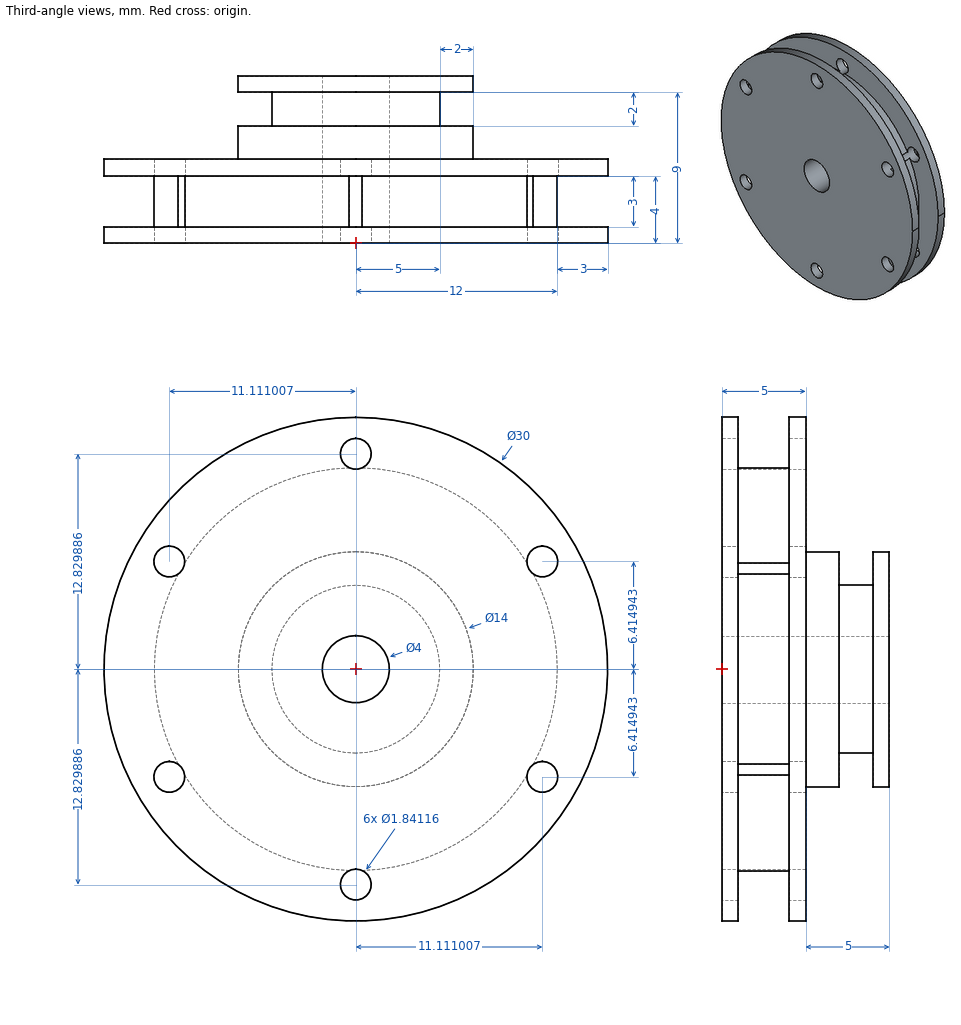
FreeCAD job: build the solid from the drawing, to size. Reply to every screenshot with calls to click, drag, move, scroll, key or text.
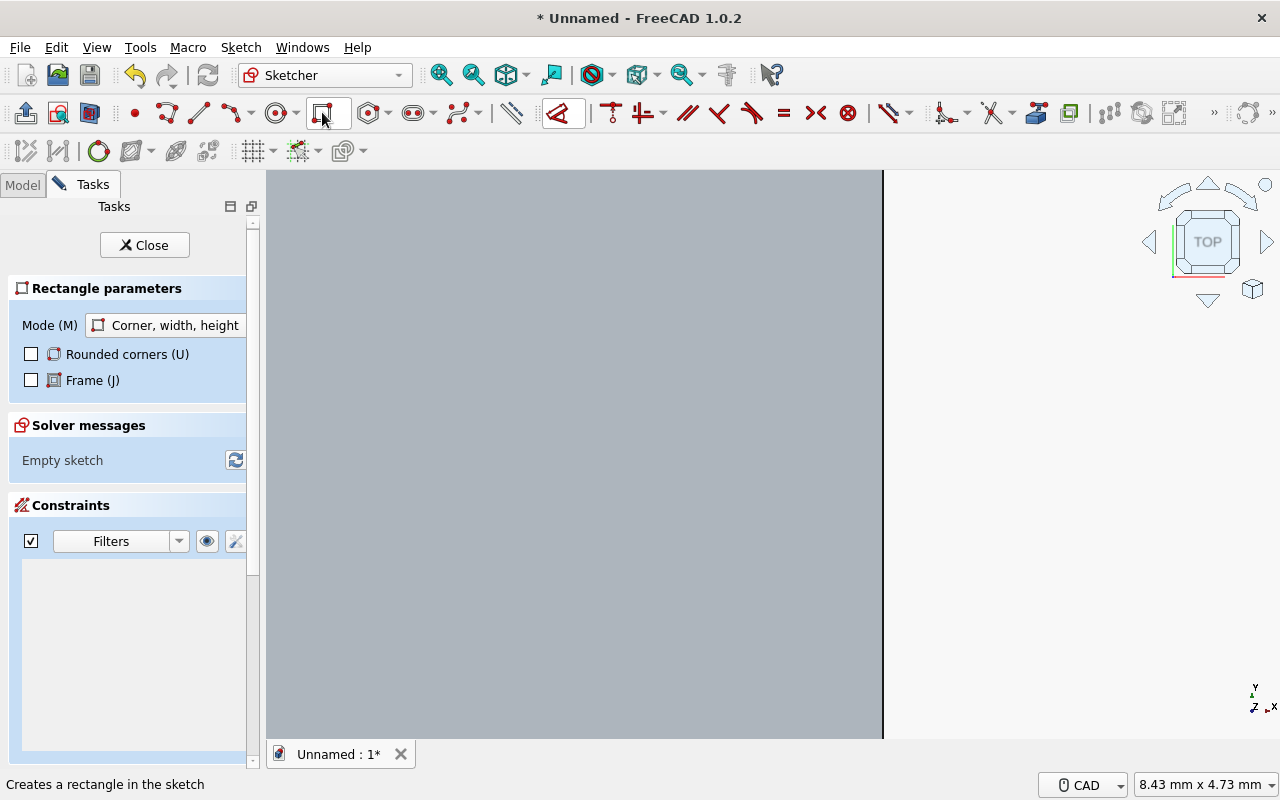
click(522, 266)
move(883, 627)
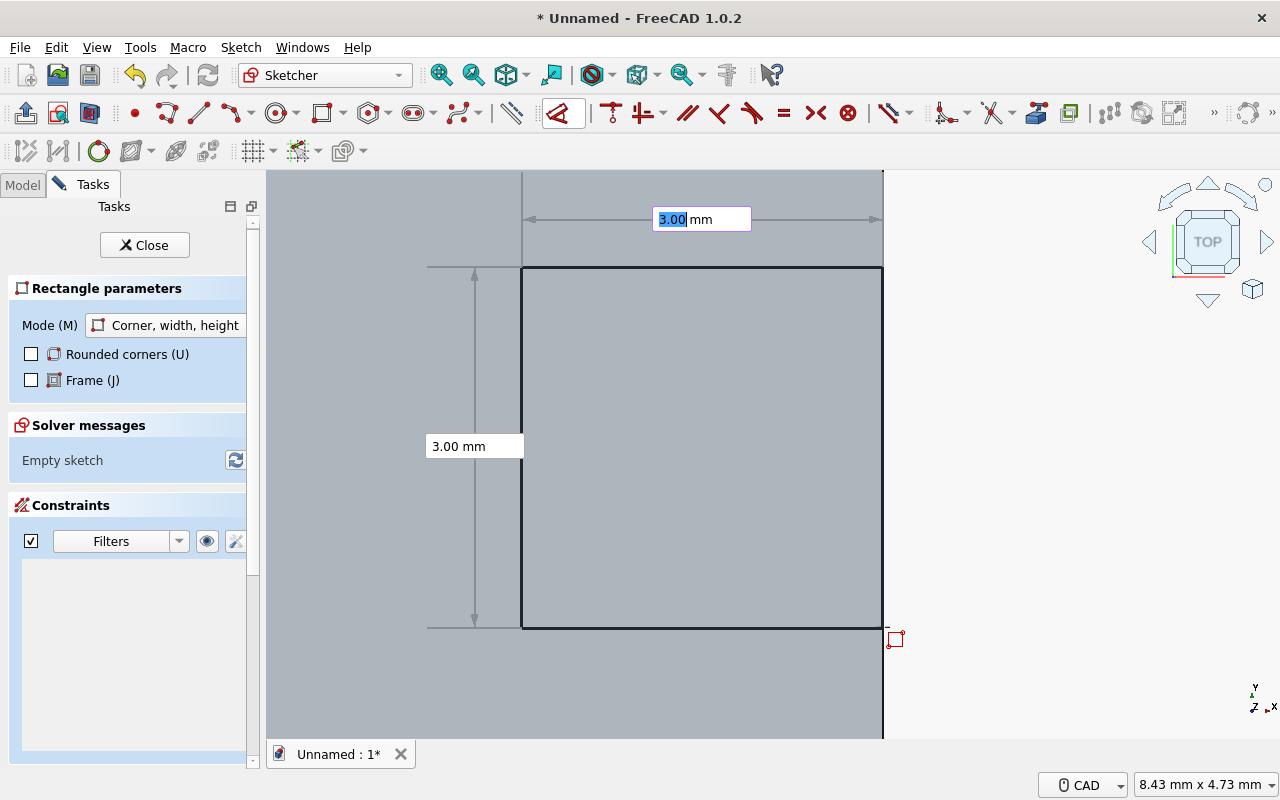
text(3)
key(Tab)
text(3)
key(Return)
key(Escape)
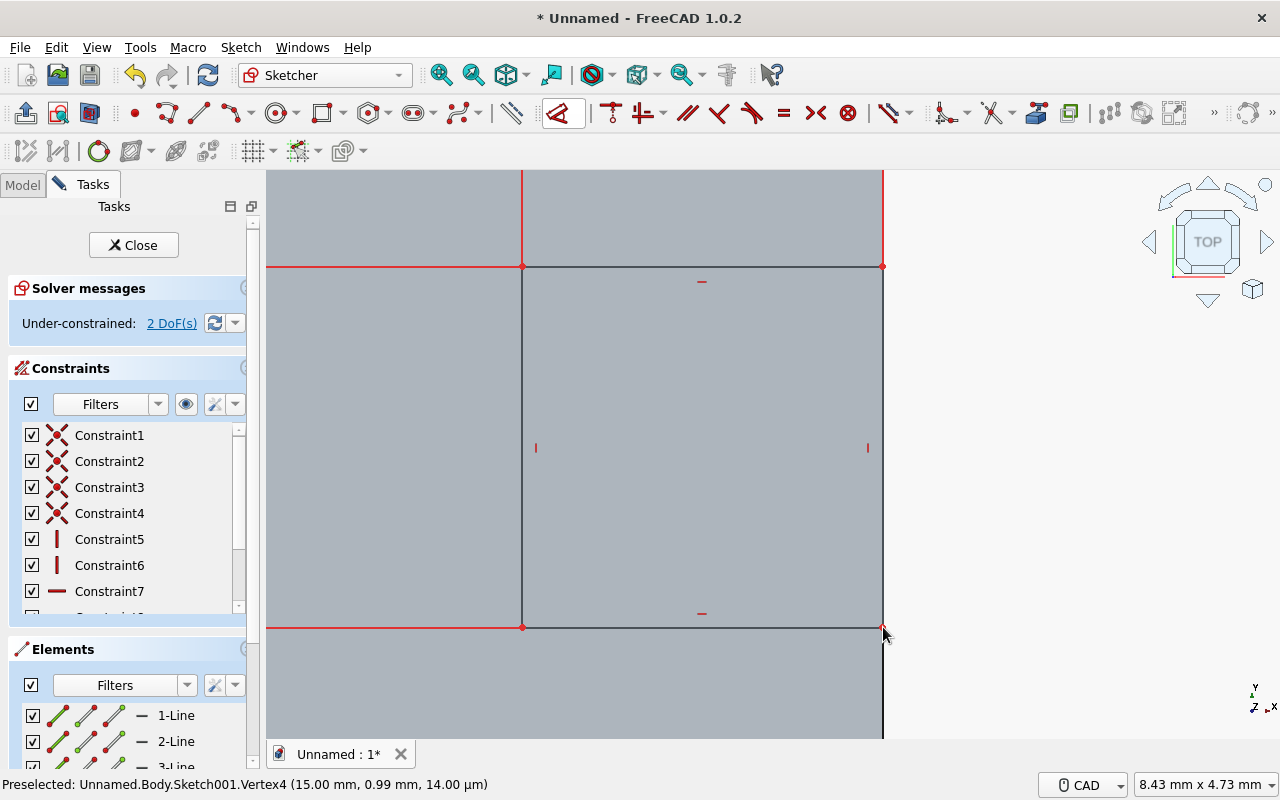
click(558, 114)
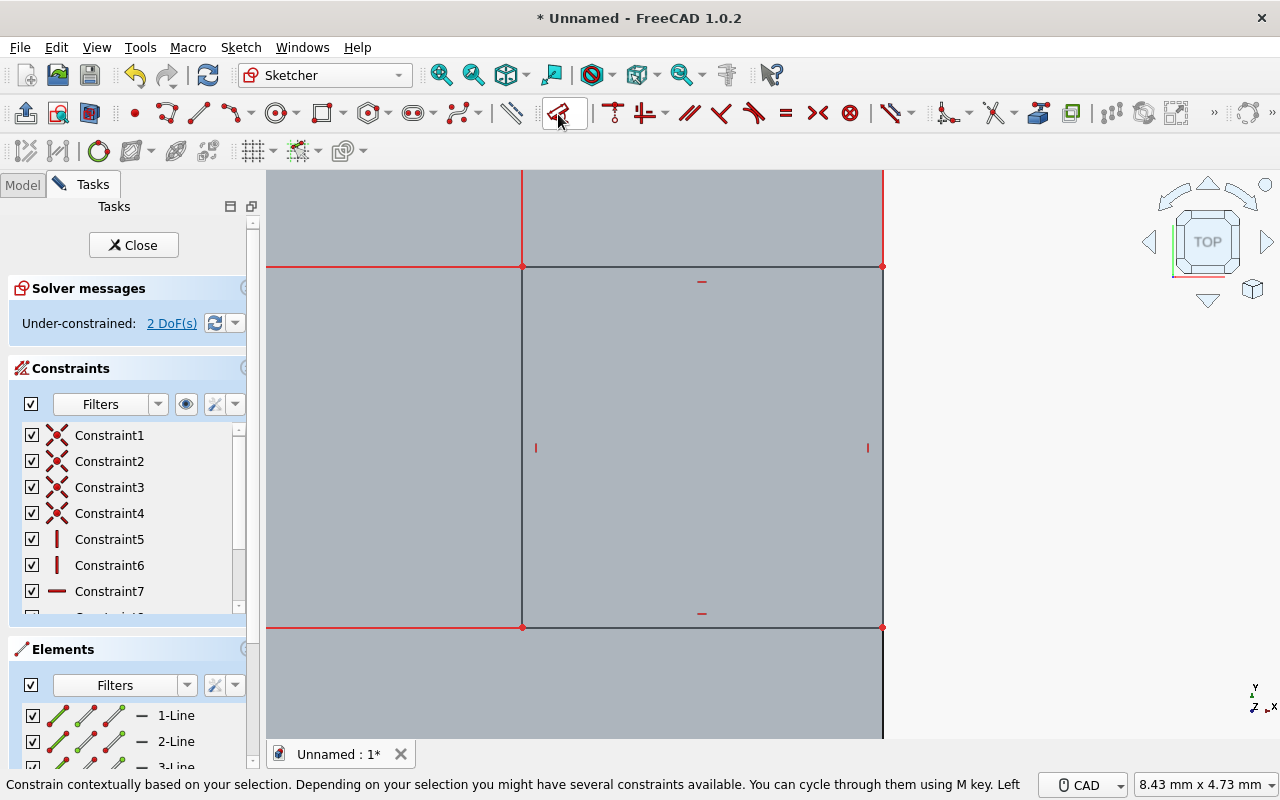
click(522, 267)
click(556, 489)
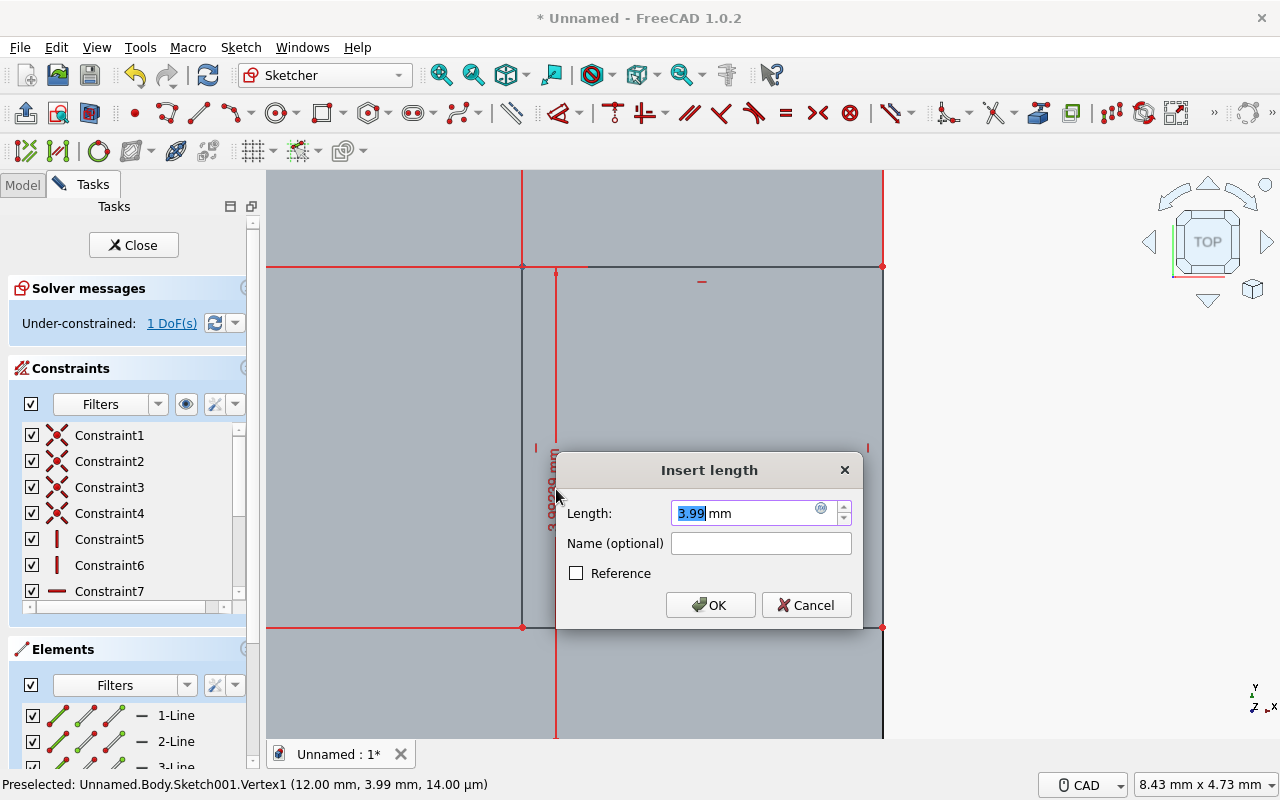
text(4)
key(Return)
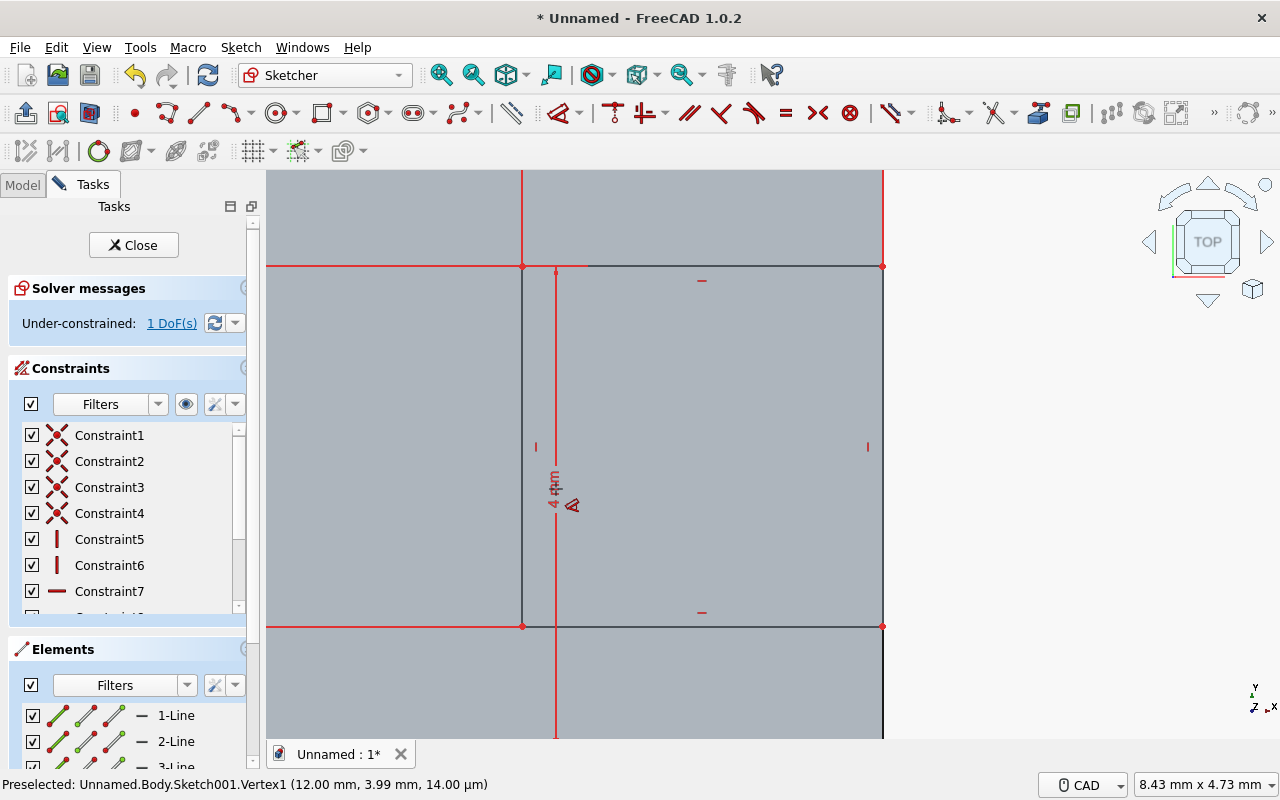
click(522, 266)
click(408, 232)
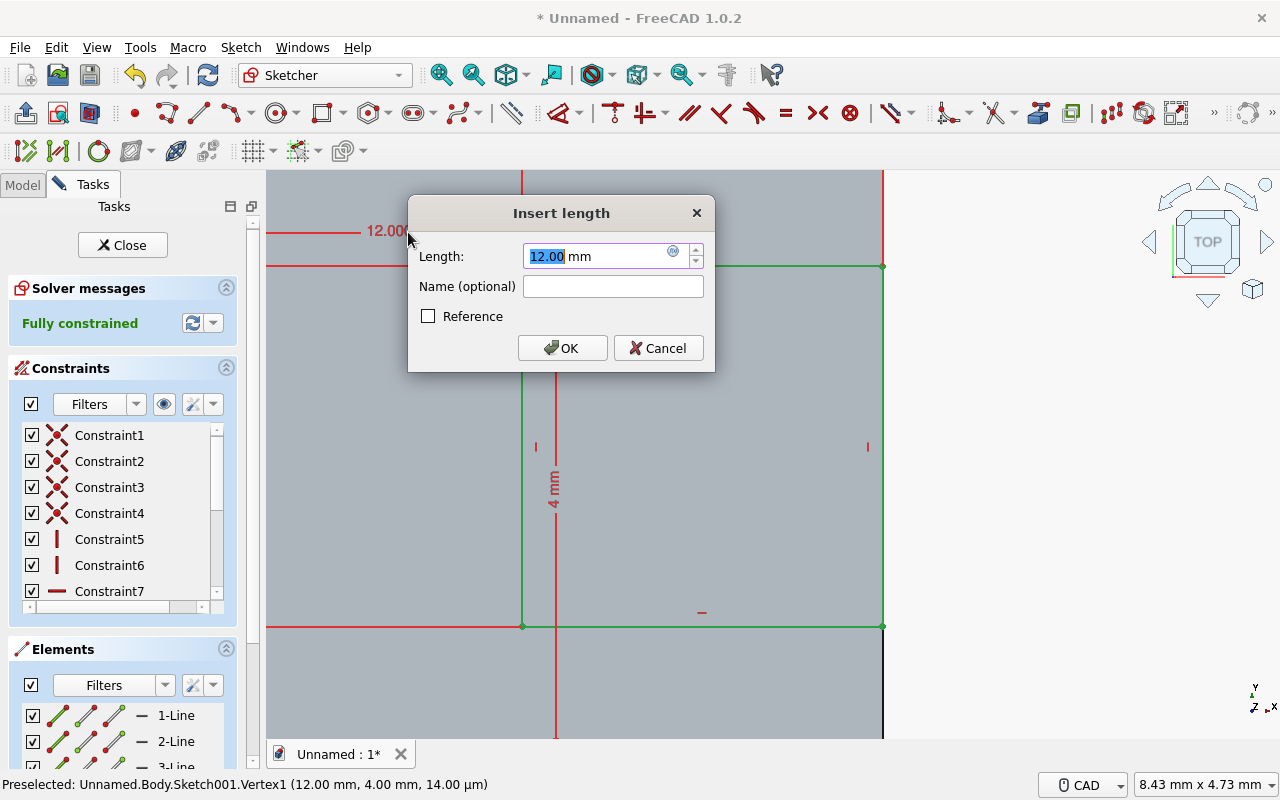
text(12)
key(Return)
key(Escape)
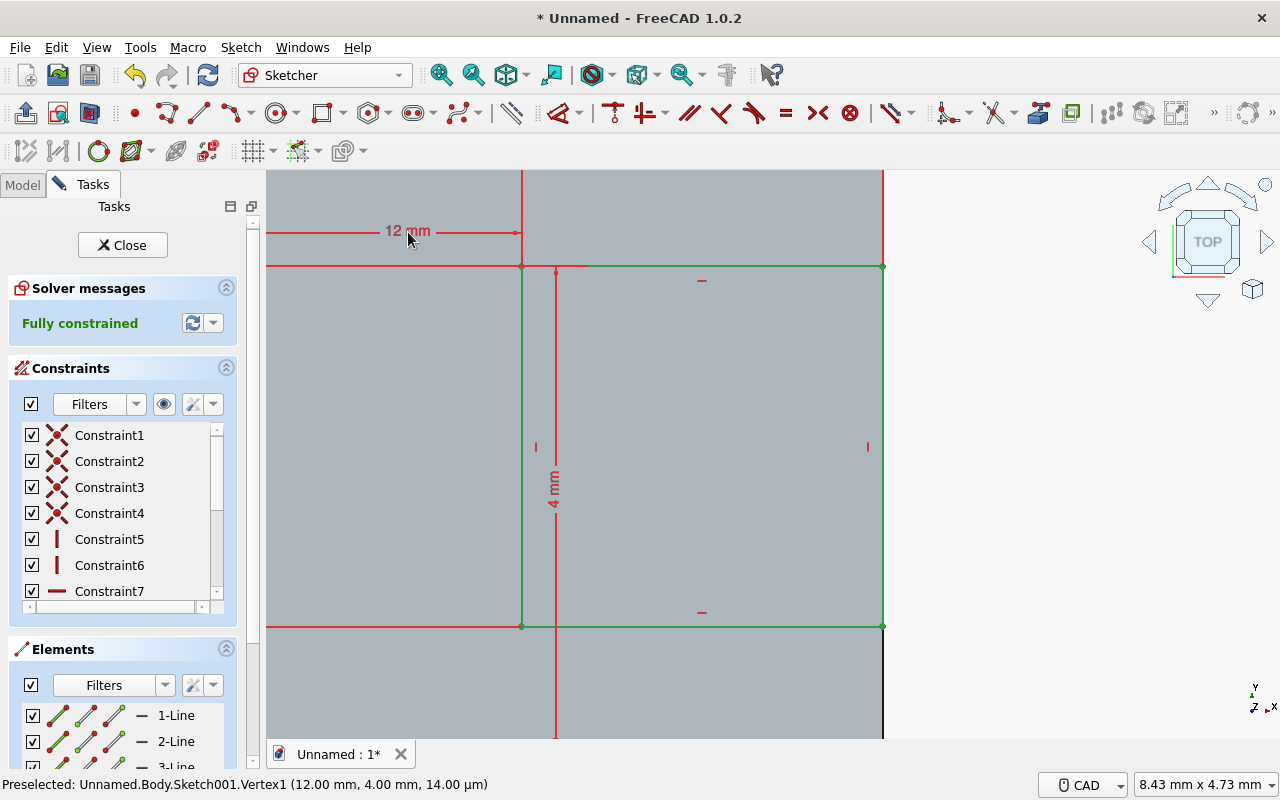
click(123, 245)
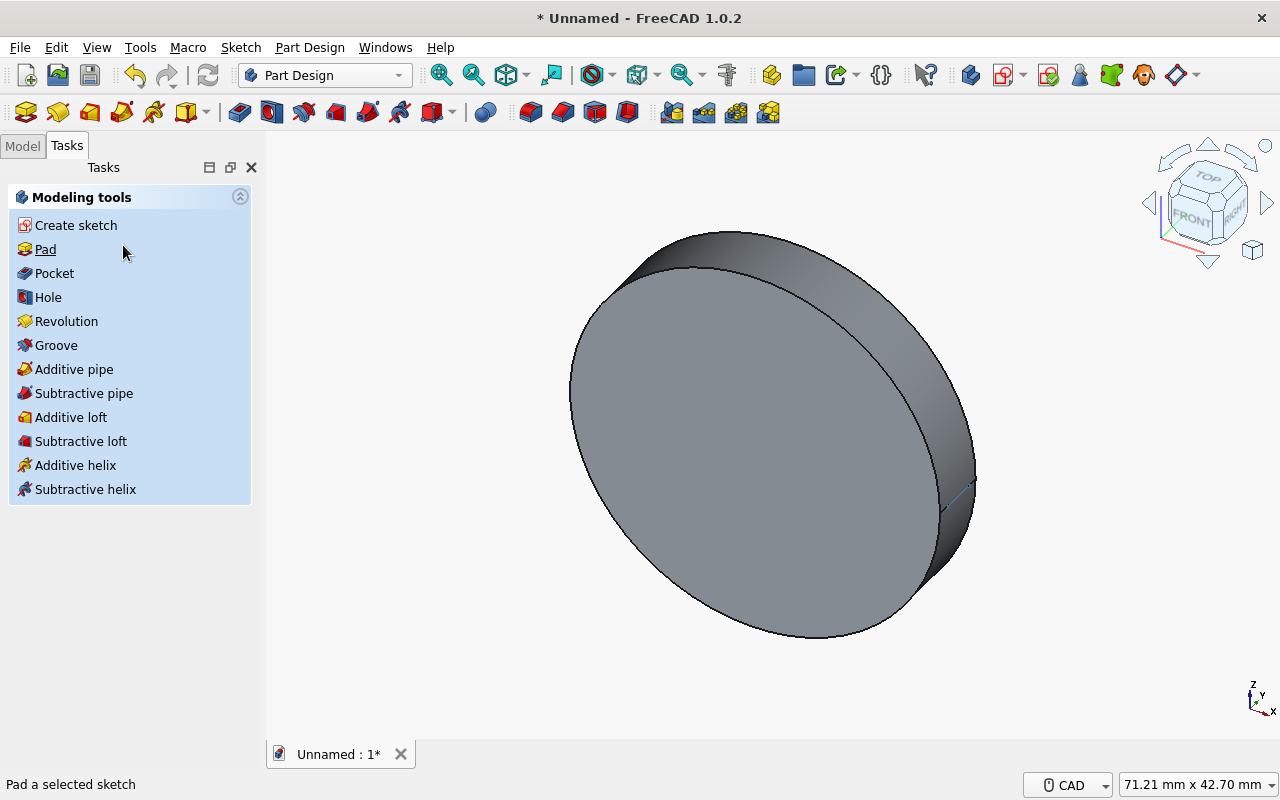
click(304, 112)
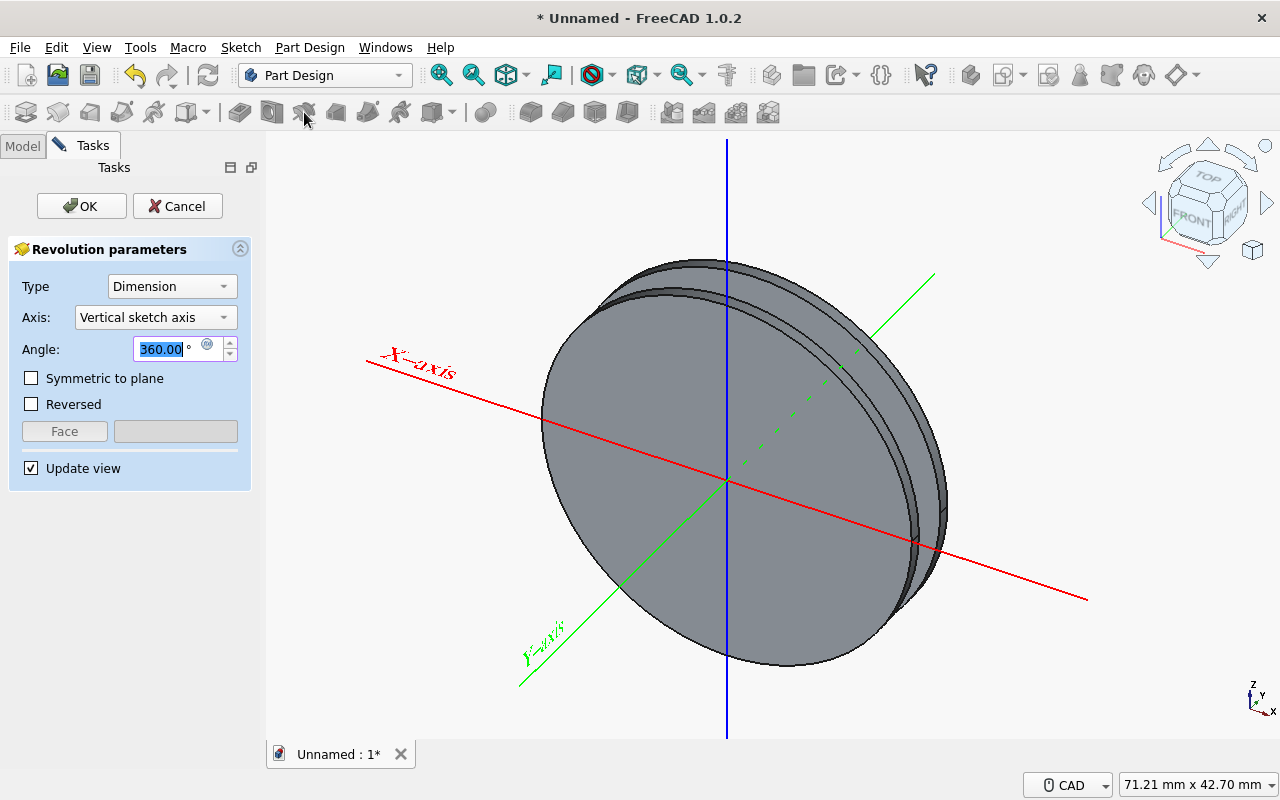
click(82, 206)